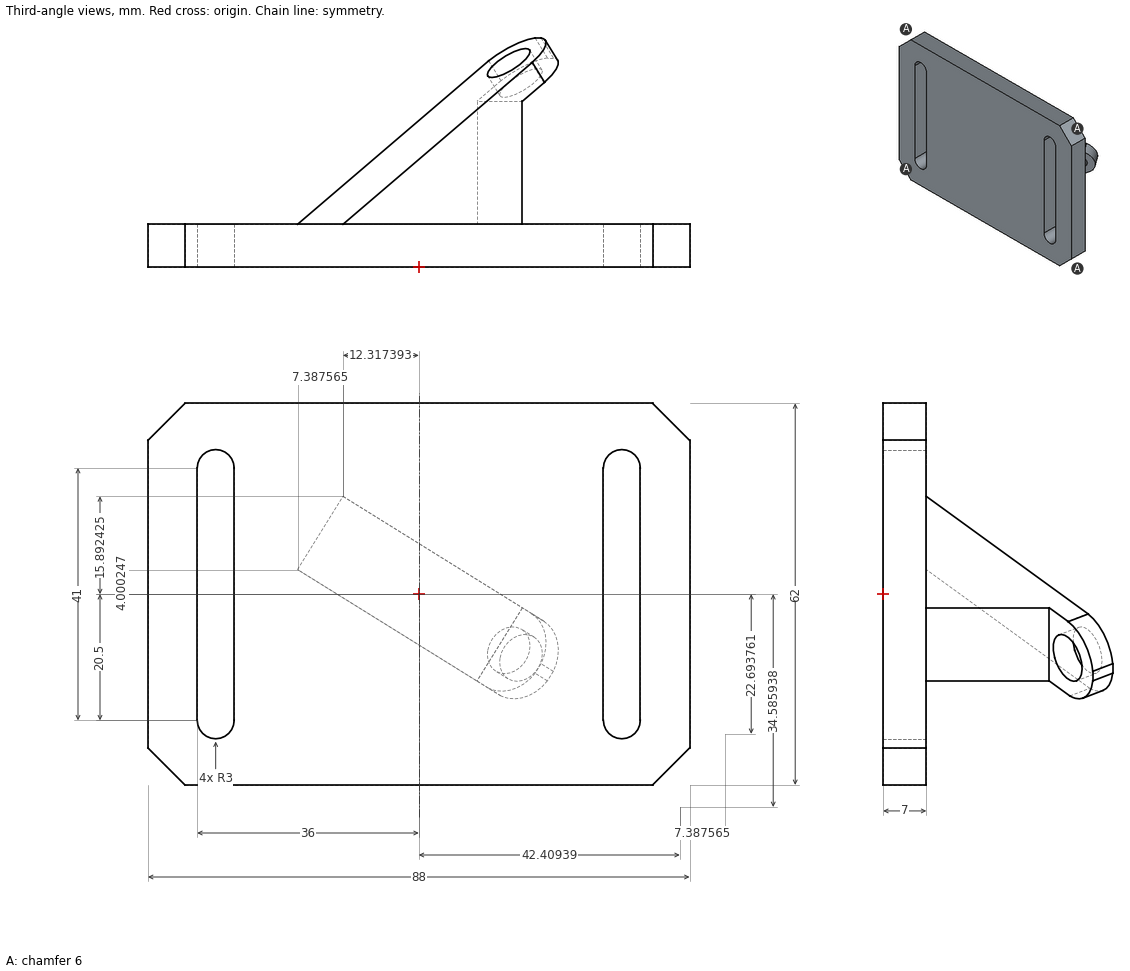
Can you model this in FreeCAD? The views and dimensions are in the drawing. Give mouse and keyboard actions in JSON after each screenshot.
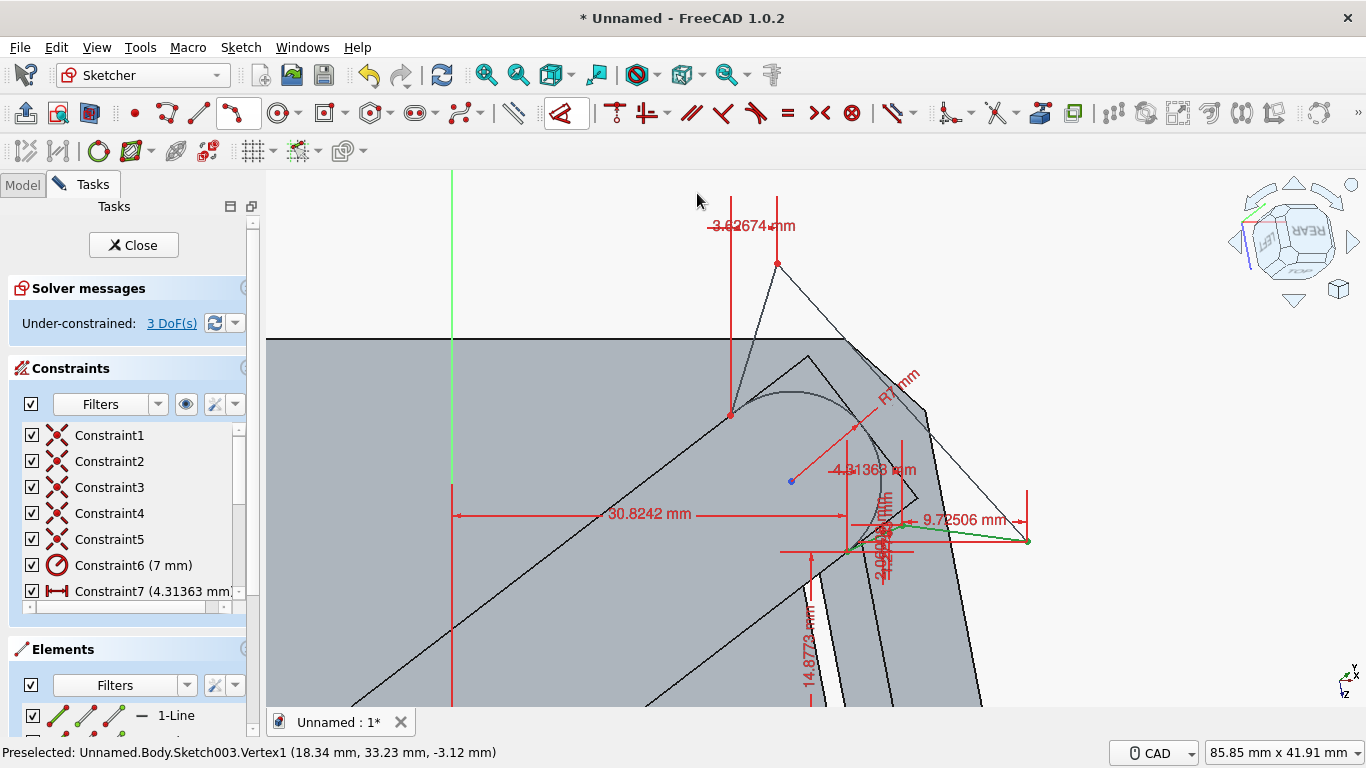
{"action": "left_click", "coordinate": [777, 264]}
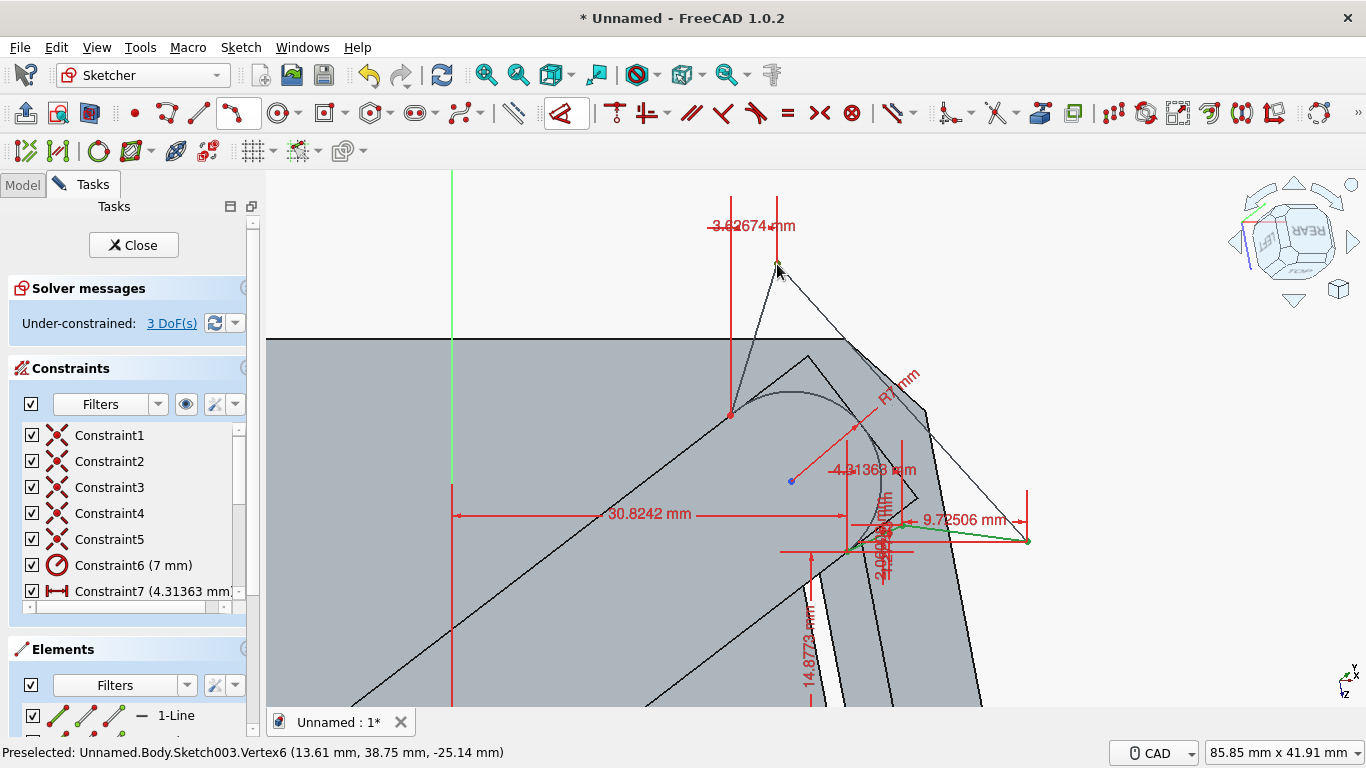
{"action": "left_click", "coordinate": [584, 114]}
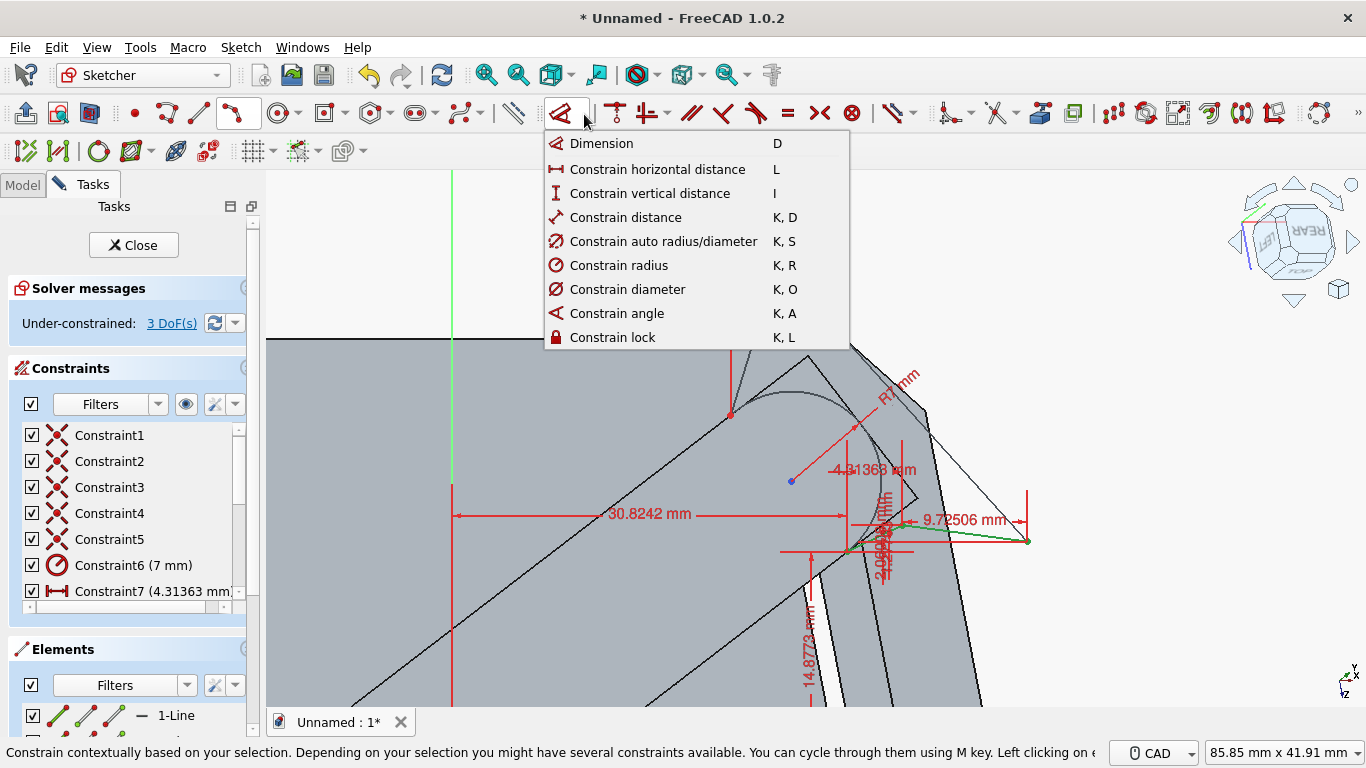
{"action": "left_click", "coordinate": [697, 169]}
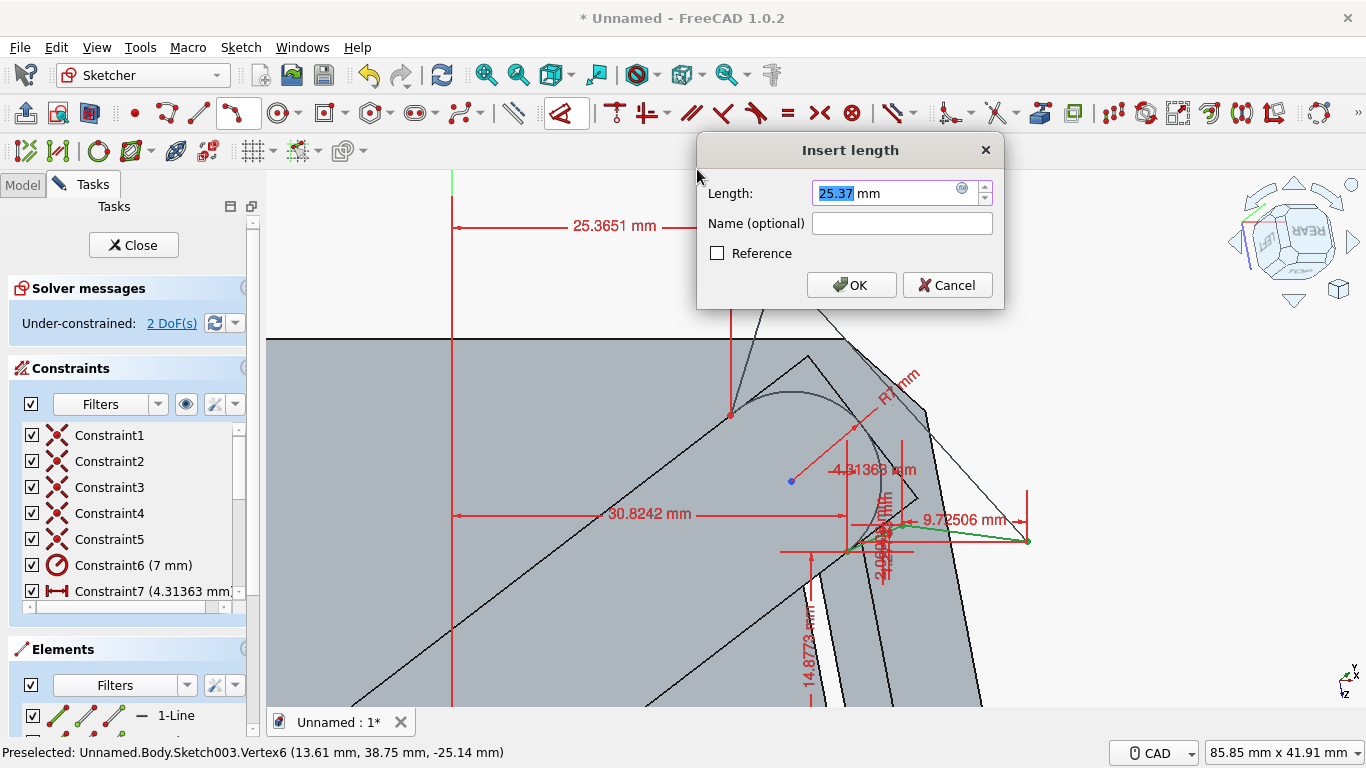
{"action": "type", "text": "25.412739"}
{"action": "key", "text": "Return"}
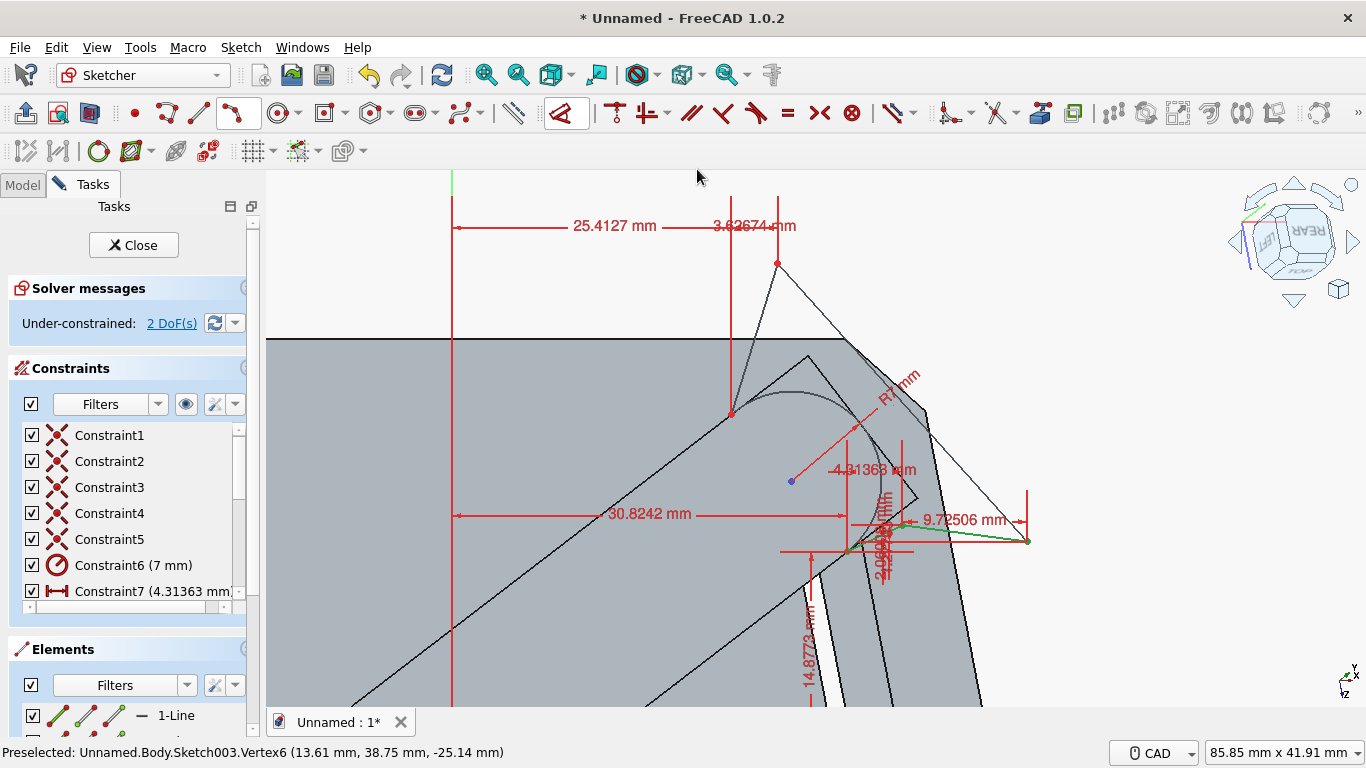
{"action": "left_click", "coordinate": [778, 264]}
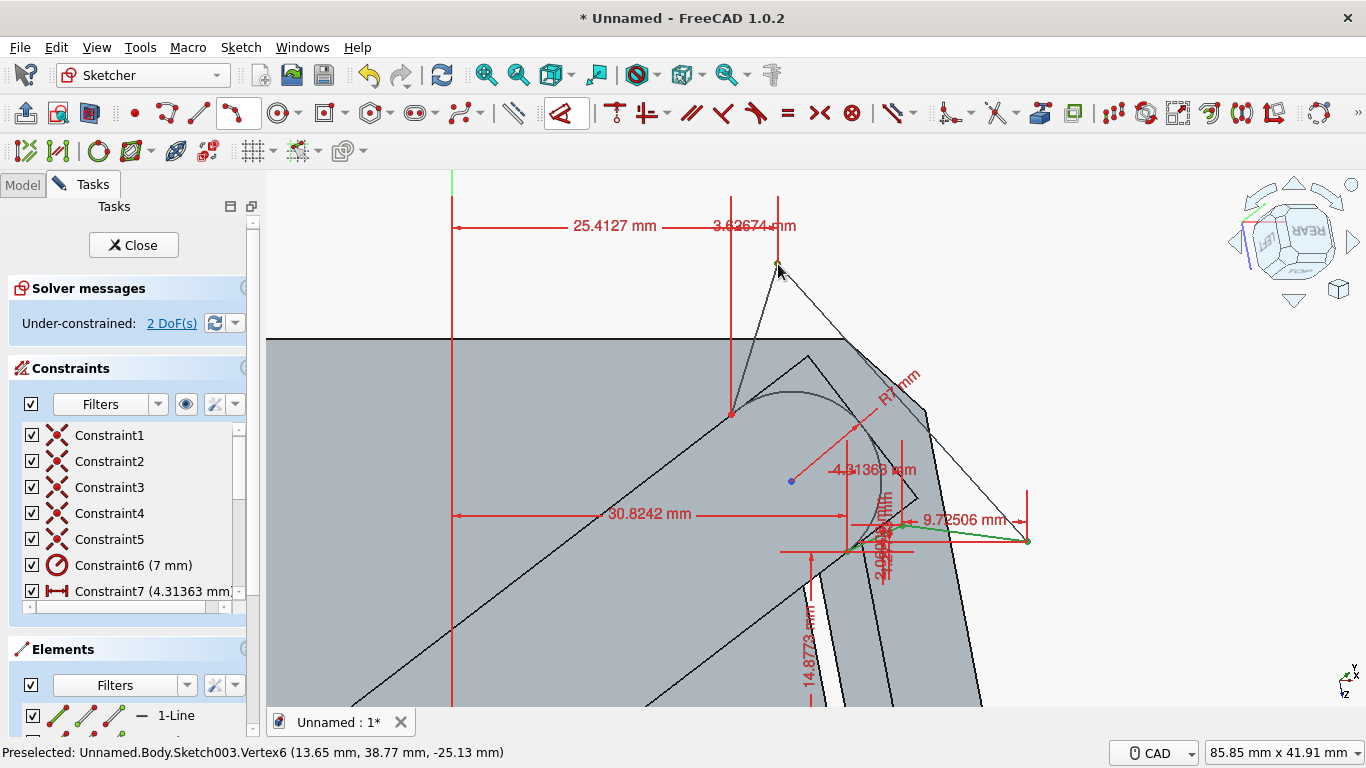
{"action": "key", "text": "i"}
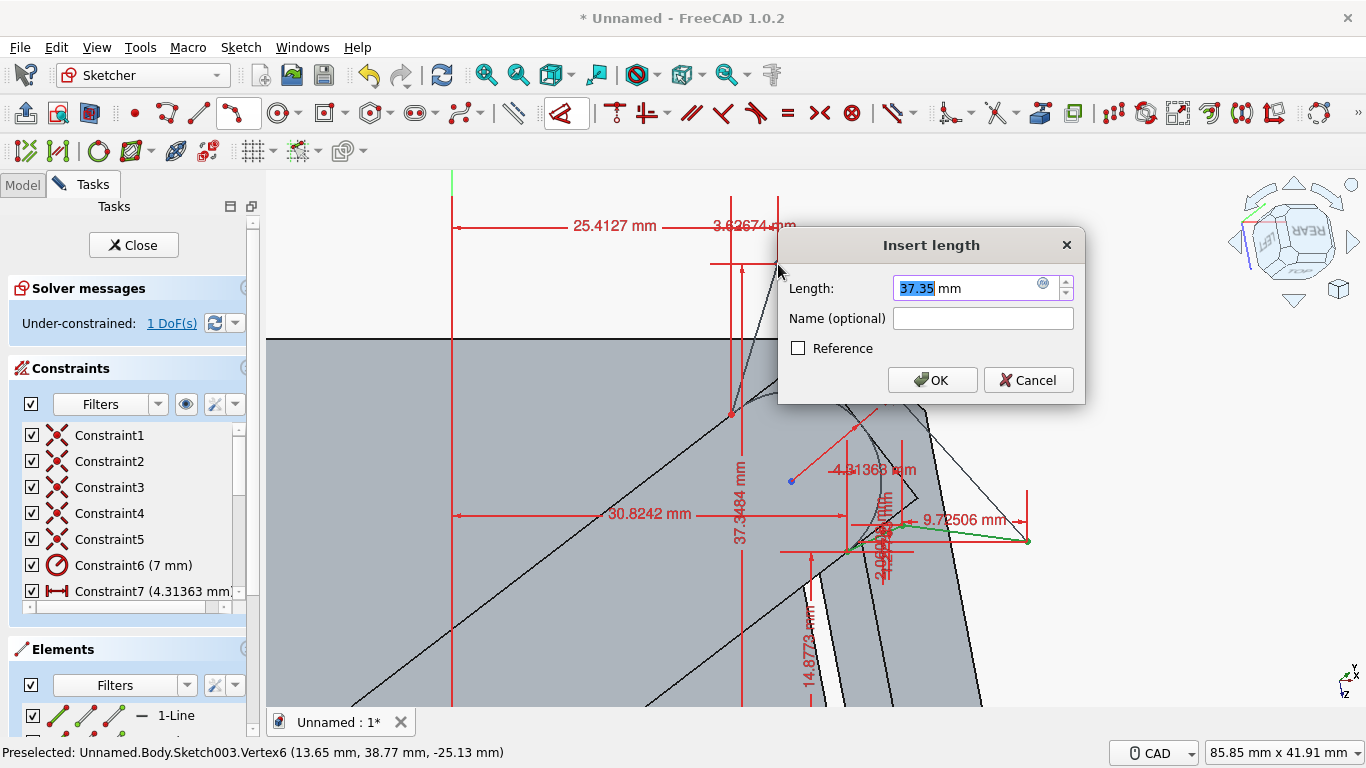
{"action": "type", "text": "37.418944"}
{"action": "key", "text": "Return"}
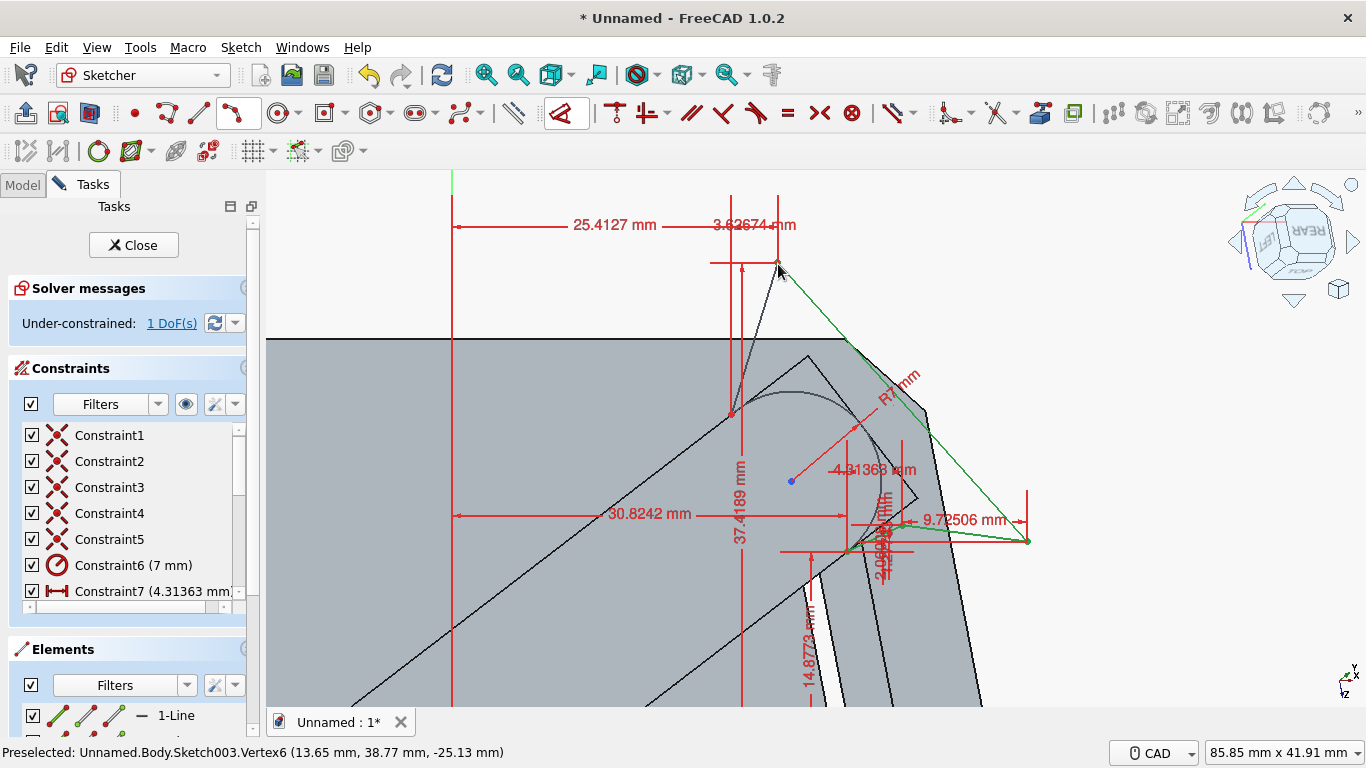
{"action": "left_click", "coordinate": [792, 481]}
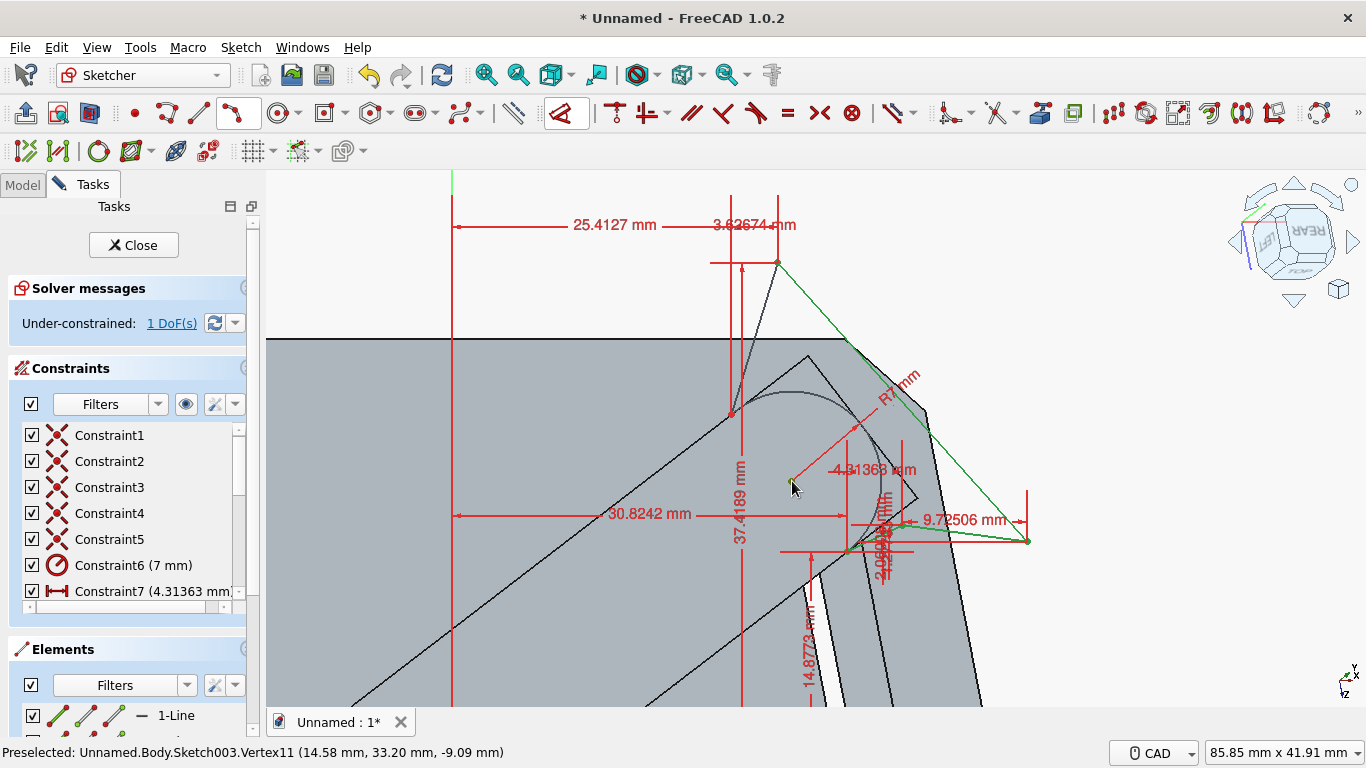
{"action": "key", "text": "l"}